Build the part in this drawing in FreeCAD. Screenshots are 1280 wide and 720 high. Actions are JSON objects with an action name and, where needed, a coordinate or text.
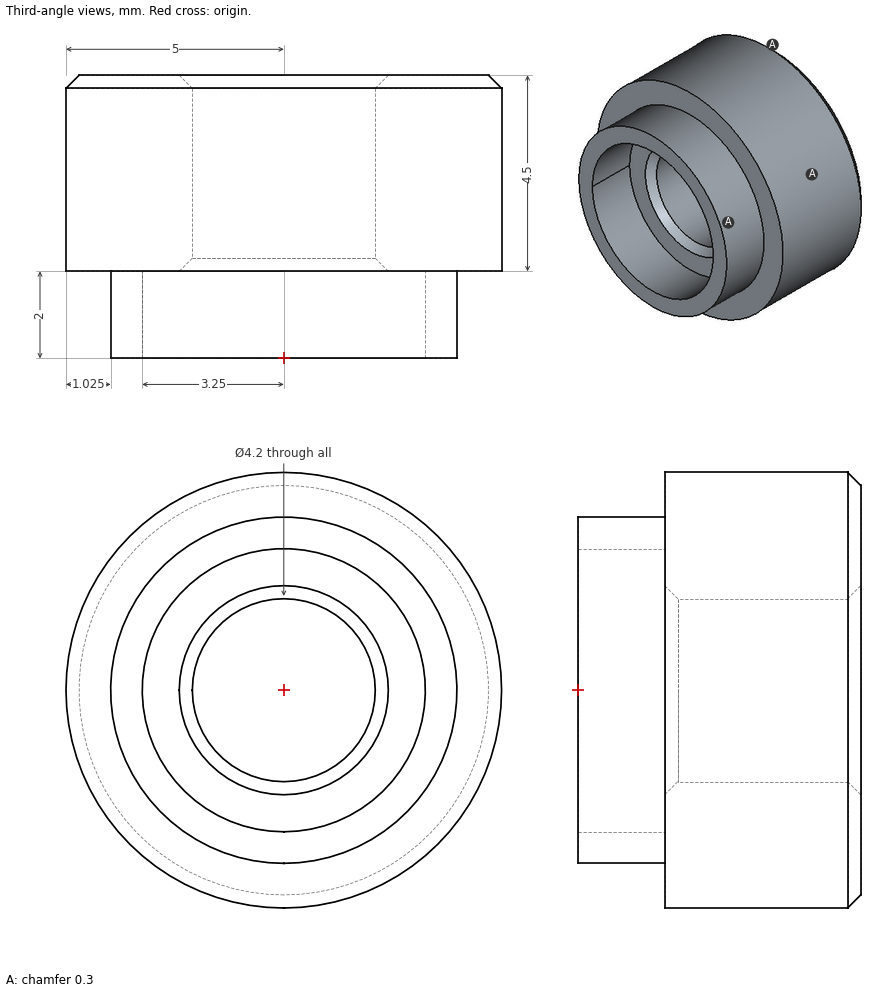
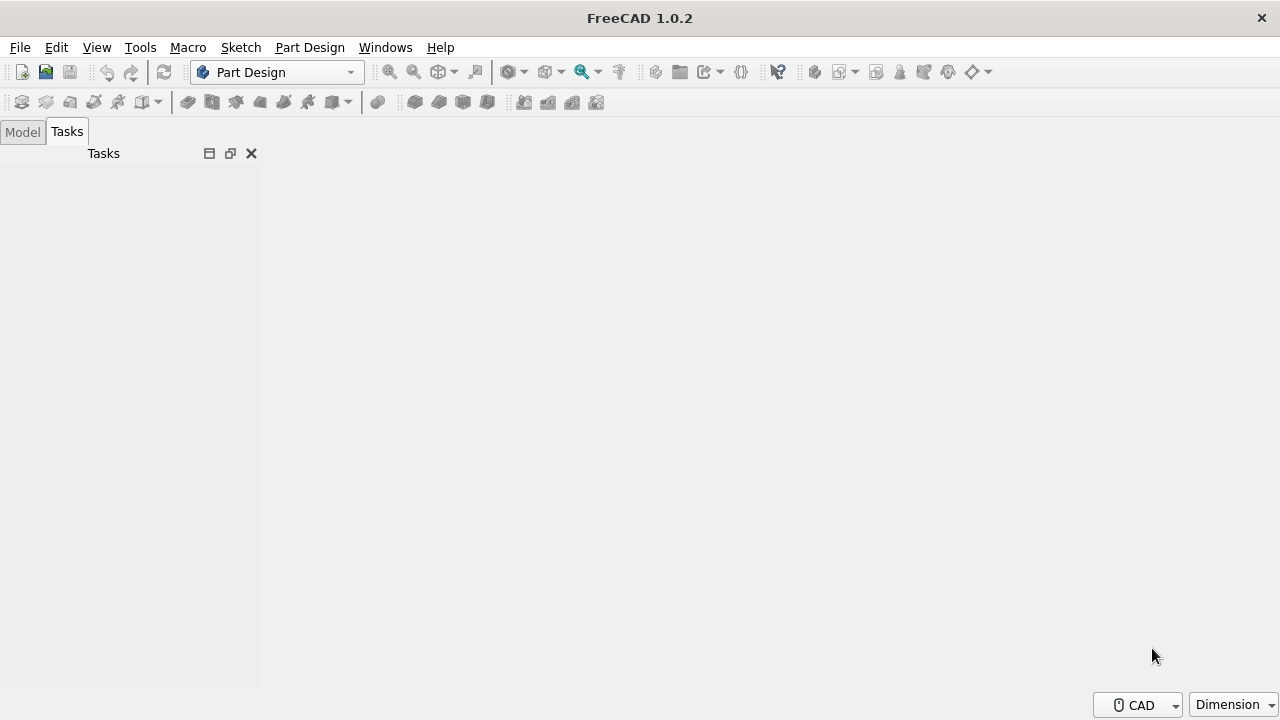
{"action": "left_click", "coordinate": [22, 72]}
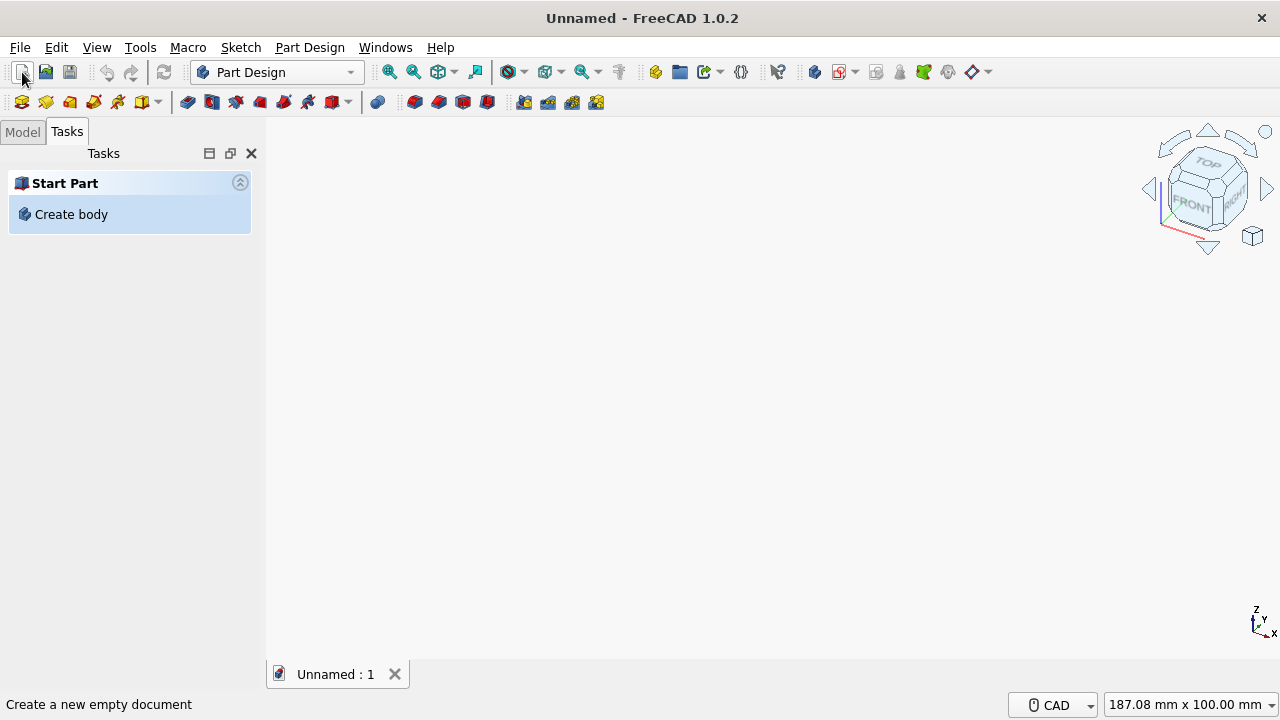
{"action": "left_click", "coordinate": [840, 72]}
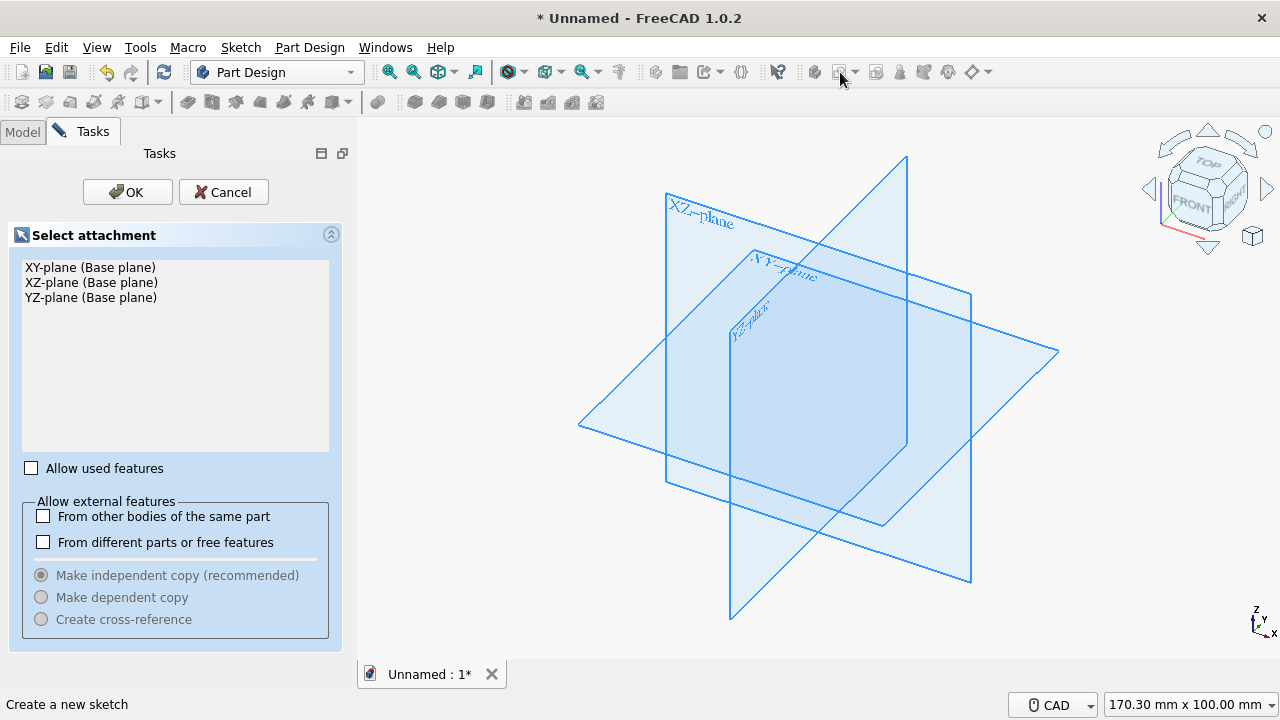
{"action": "left_click", "coordinate": [82, 268]}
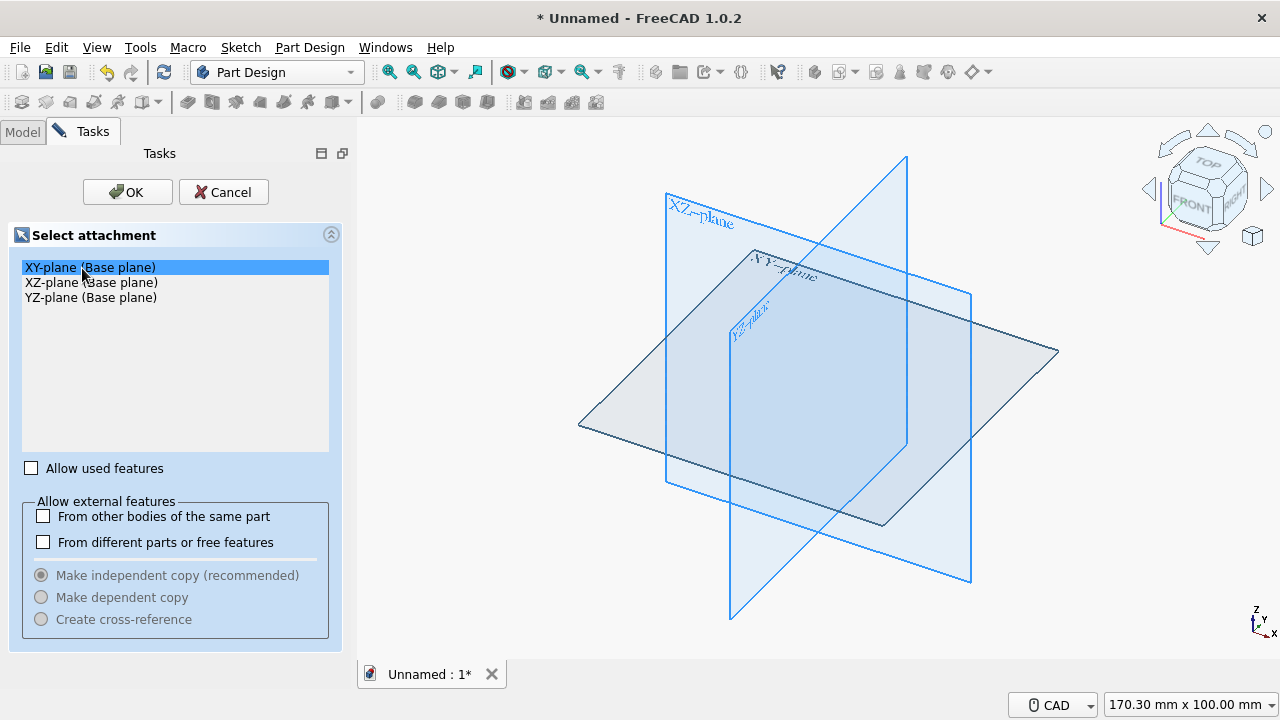
{"action": "left_click", "coordinate": [128, 192]}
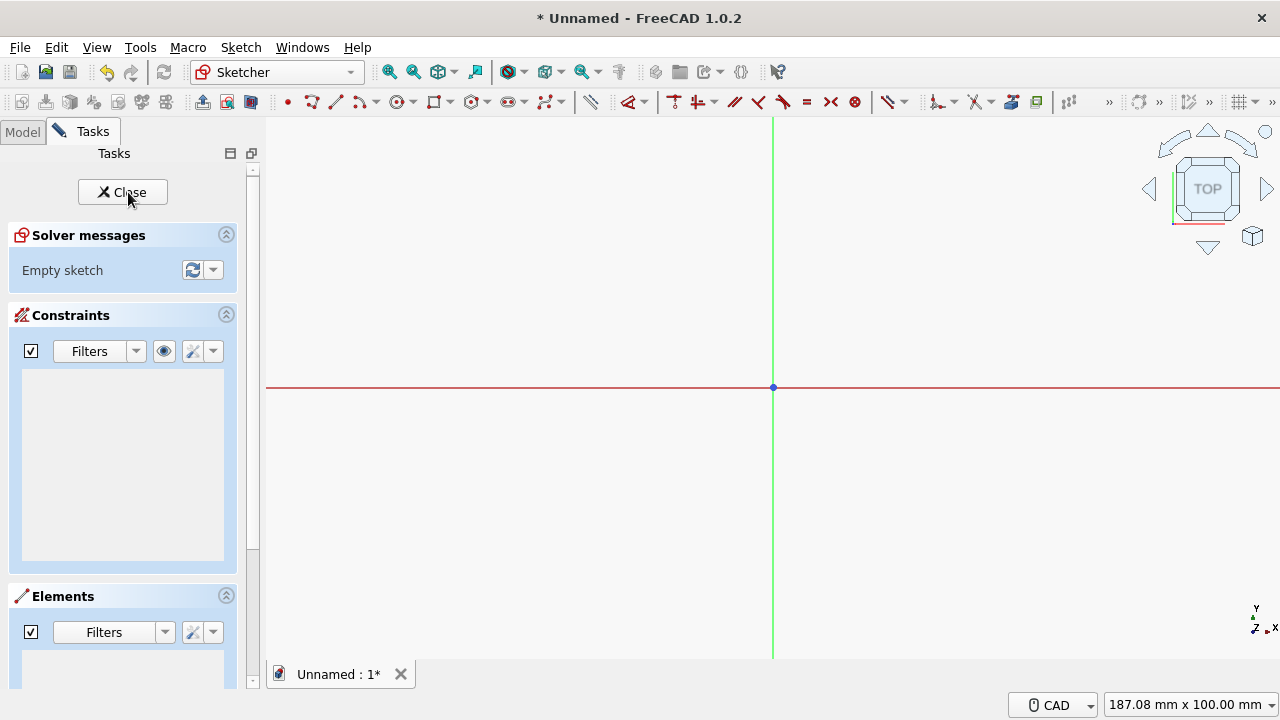
{"action": "scroll", "coordinate": [766, 368], "scroll_direction": "up", "scroll_amount": 11}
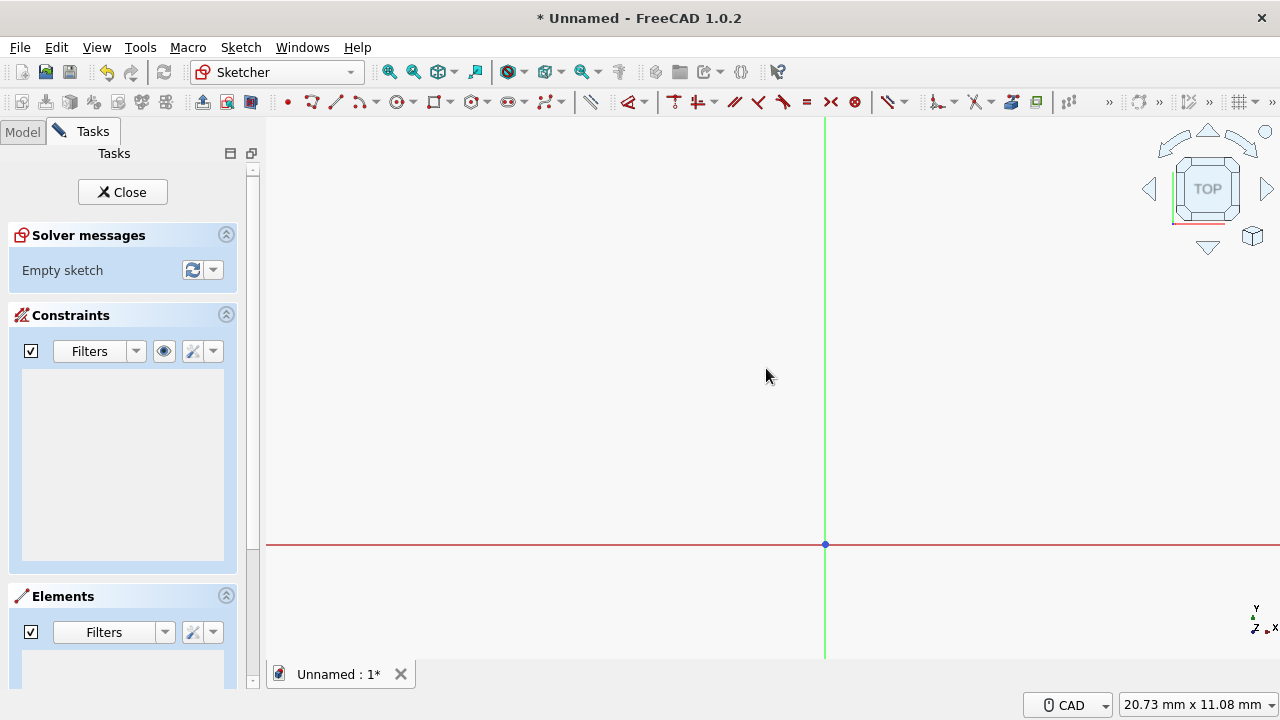
{"action": "left_click", "coordinate": [312, 102]}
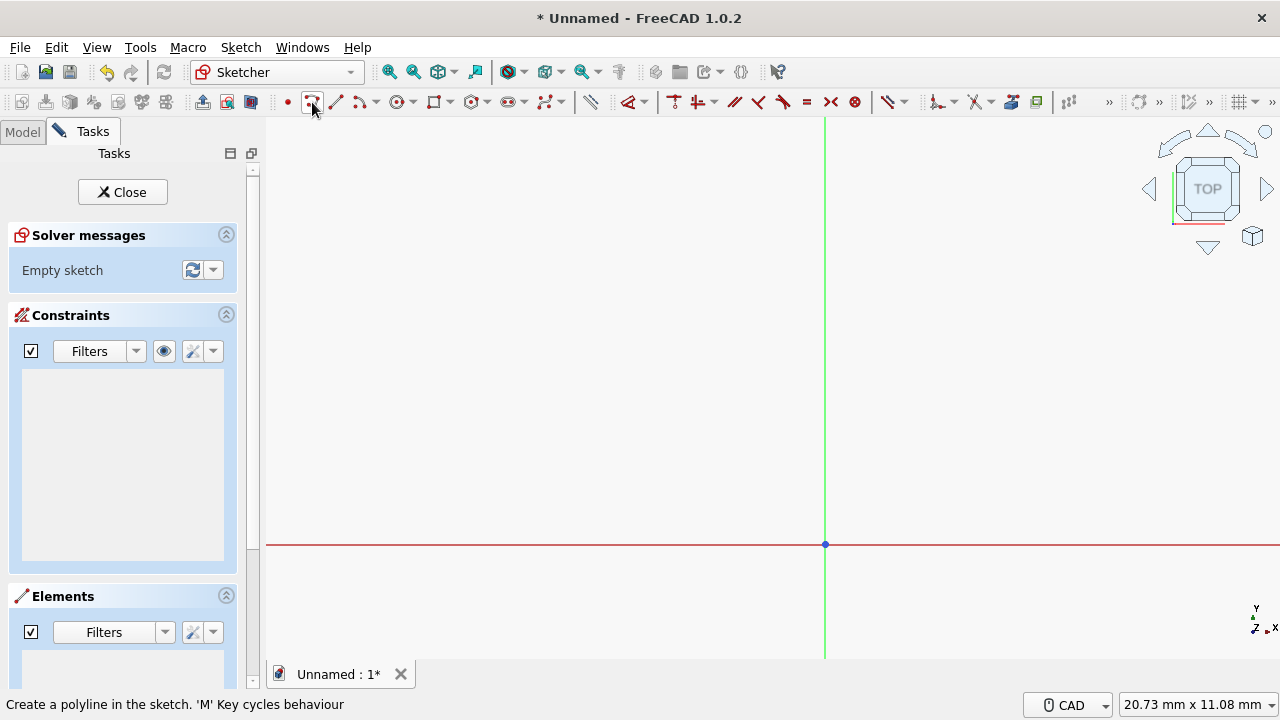
{"action": "left_click", "coordinate": [825, 447]}
{"action": "left_click", "coordinate": [816, 227]}
{"action": "left_click", "coordinate": [581, 227]}
{"action": "left_click", "coordinate": [581, 447]}
{"action": "left_click", "coordinate": [631, 447]}
{"action": "left_click", "coordinate": [631, 545]}
{"action": "left_click", "coordinate": [666, 536]}
{"action": "left_click", "coordinate": [666, 447]}
{"action": "left_click", "coordinate": [825, 448]}
{"action": "key", "text": "Escape"}
{"action": "key", "text": "Escape"}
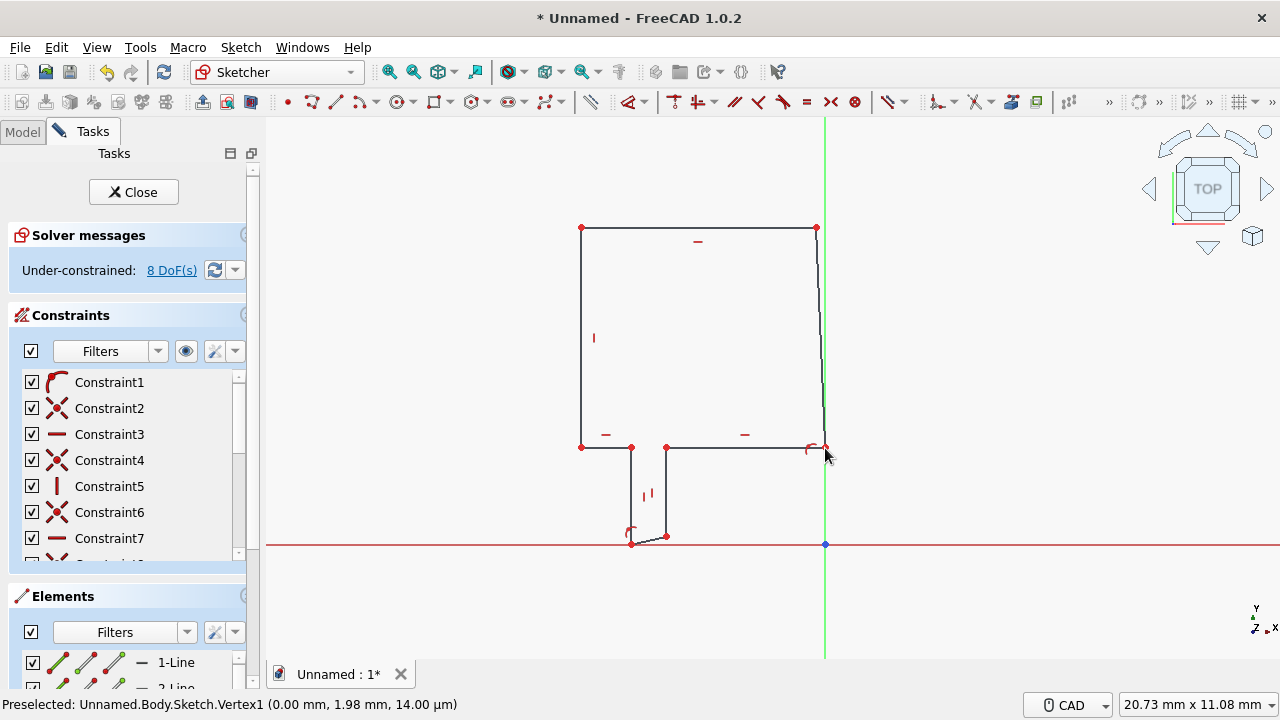
{"action": "left_click", "coordinate": [822, 382]}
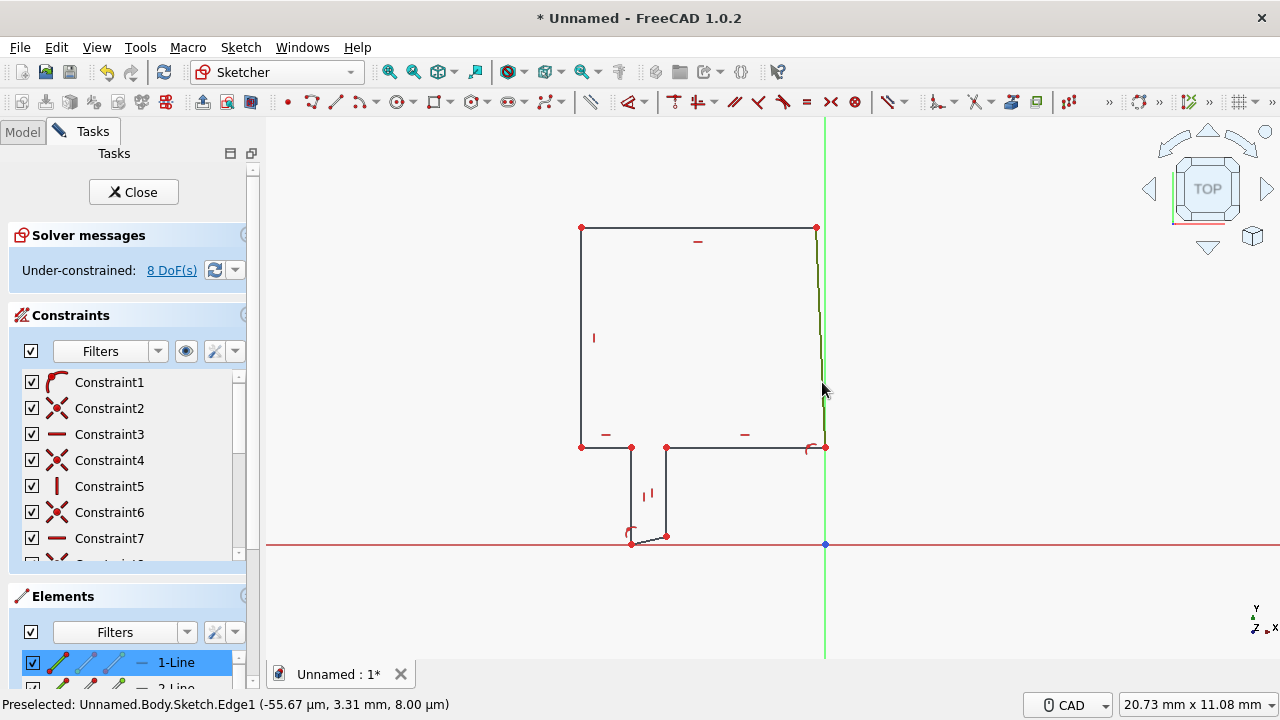
{"action": "left_click", "coordinate": [716, 102]}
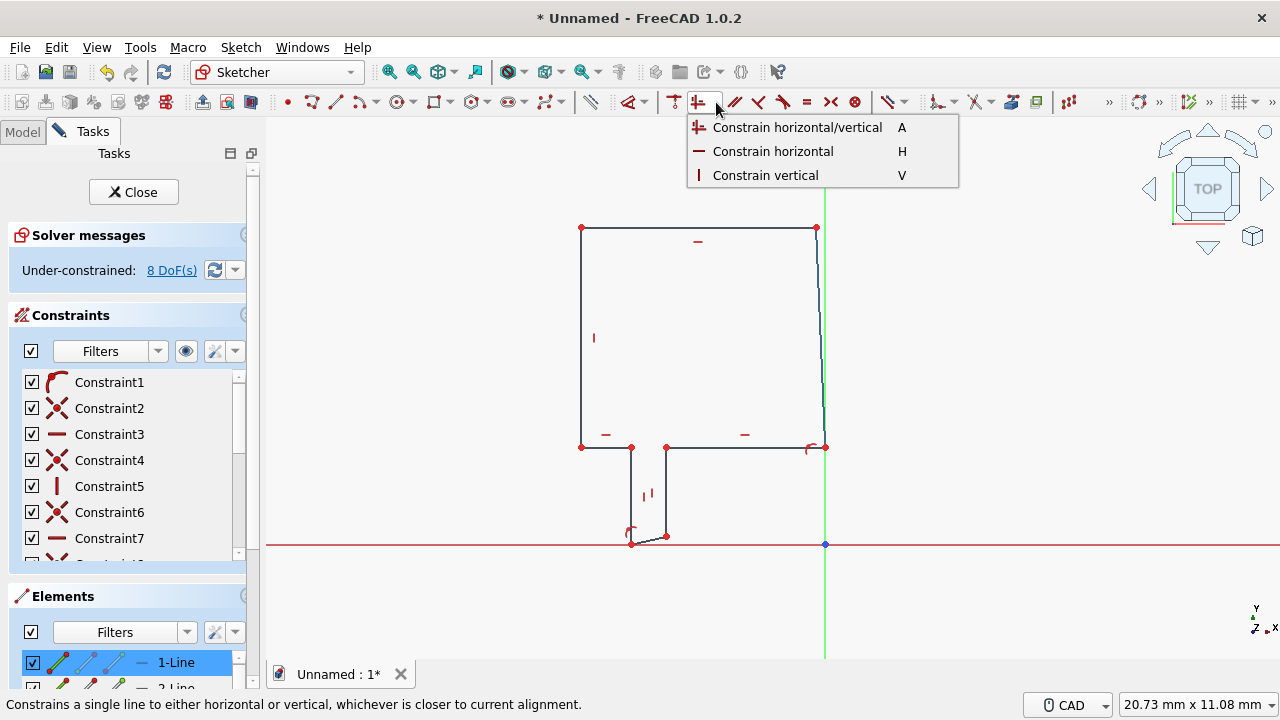
{"action": "left_click", "coordinate": [823, 175]}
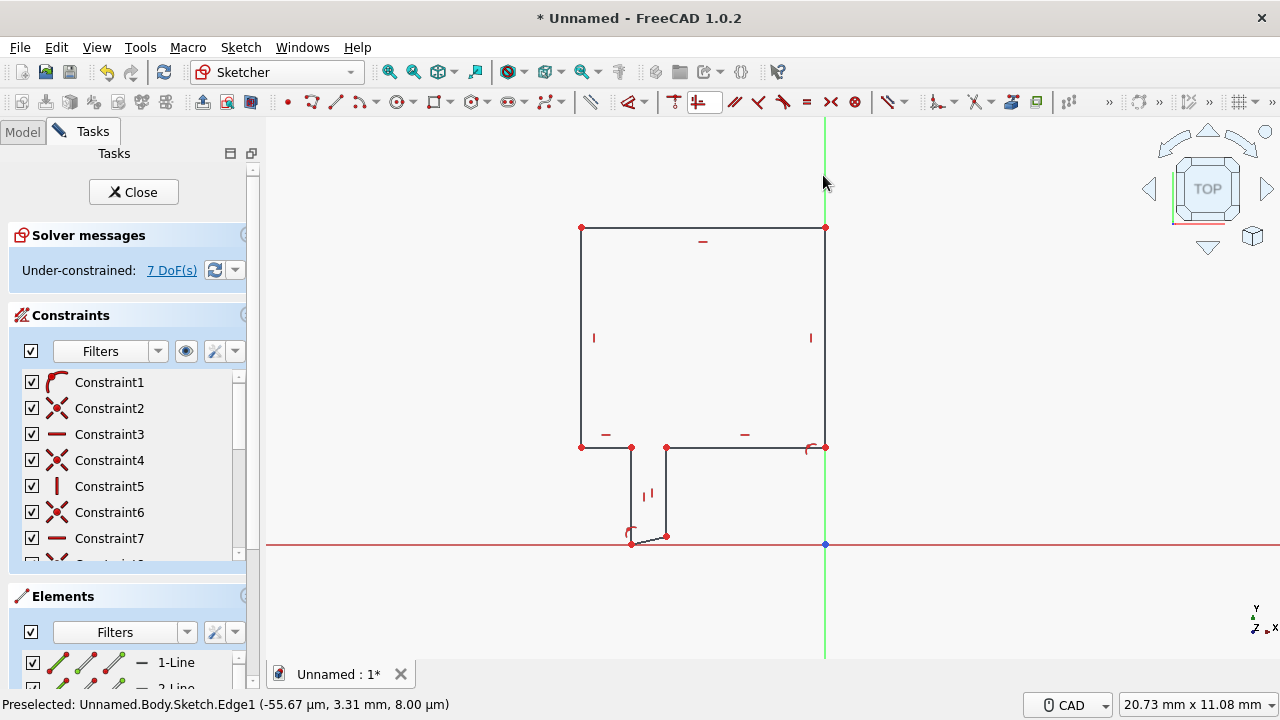
{"action": "scroll", "coordinate": [641, 542], "scroll_direction": "up", "scroll_amount": 2}